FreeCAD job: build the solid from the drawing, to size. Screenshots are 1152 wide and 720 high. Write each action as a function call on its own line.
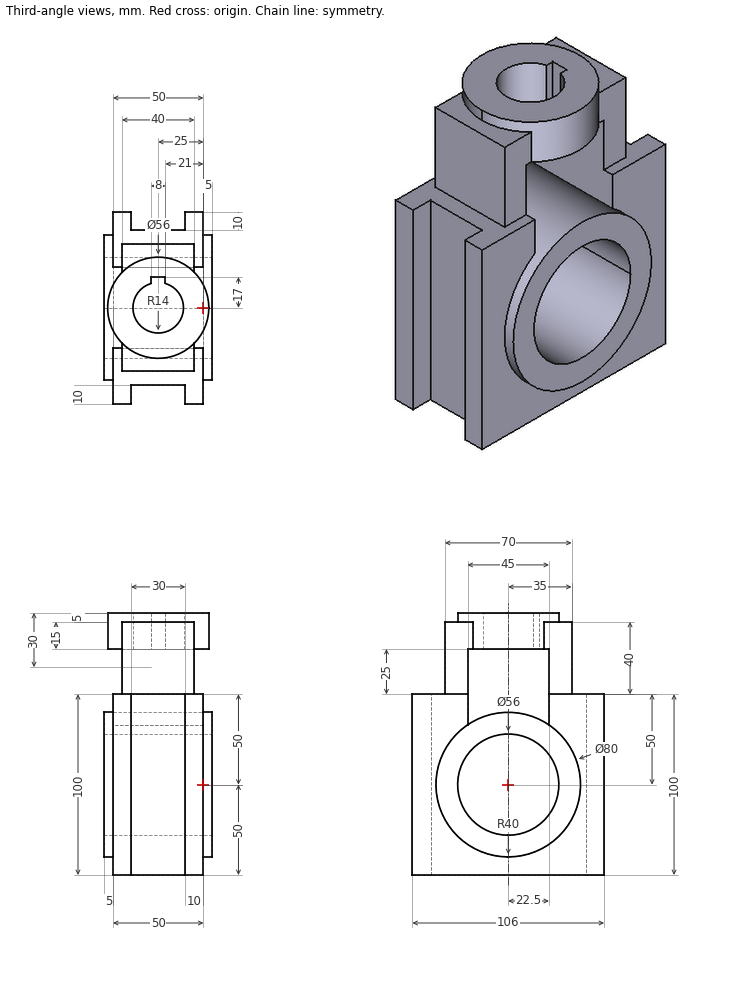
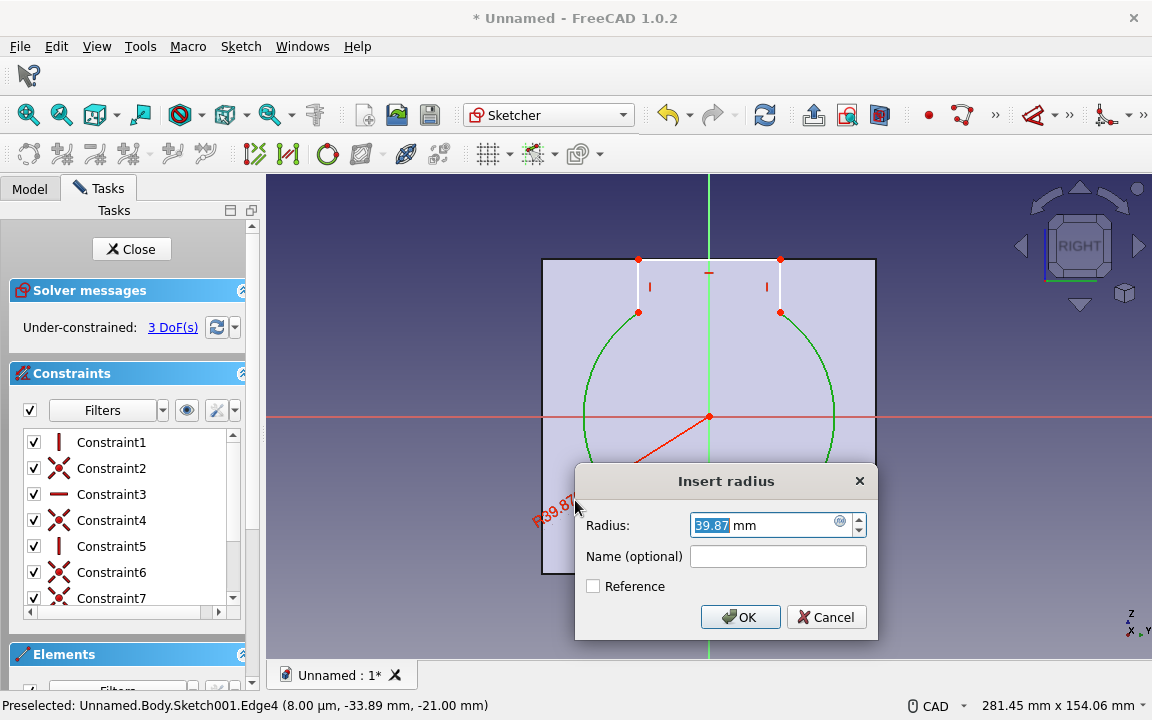
text(40)
key(Return)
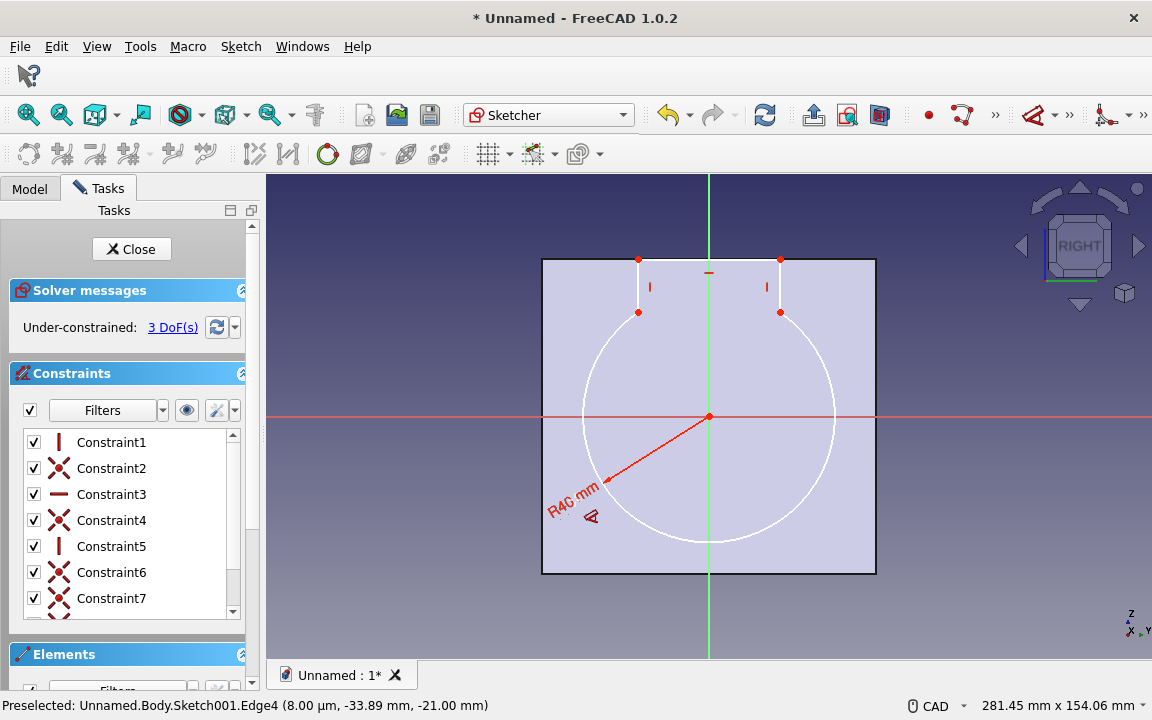
click(737, 260)
click(676, 226)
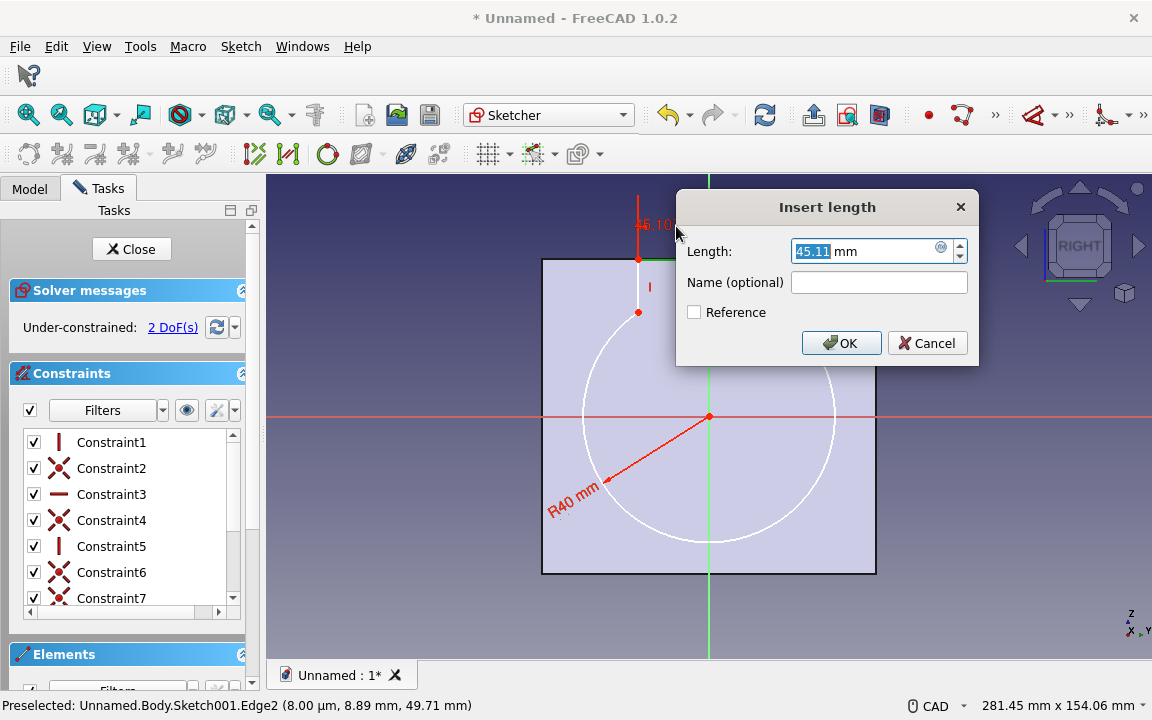
text(45)
key(Return)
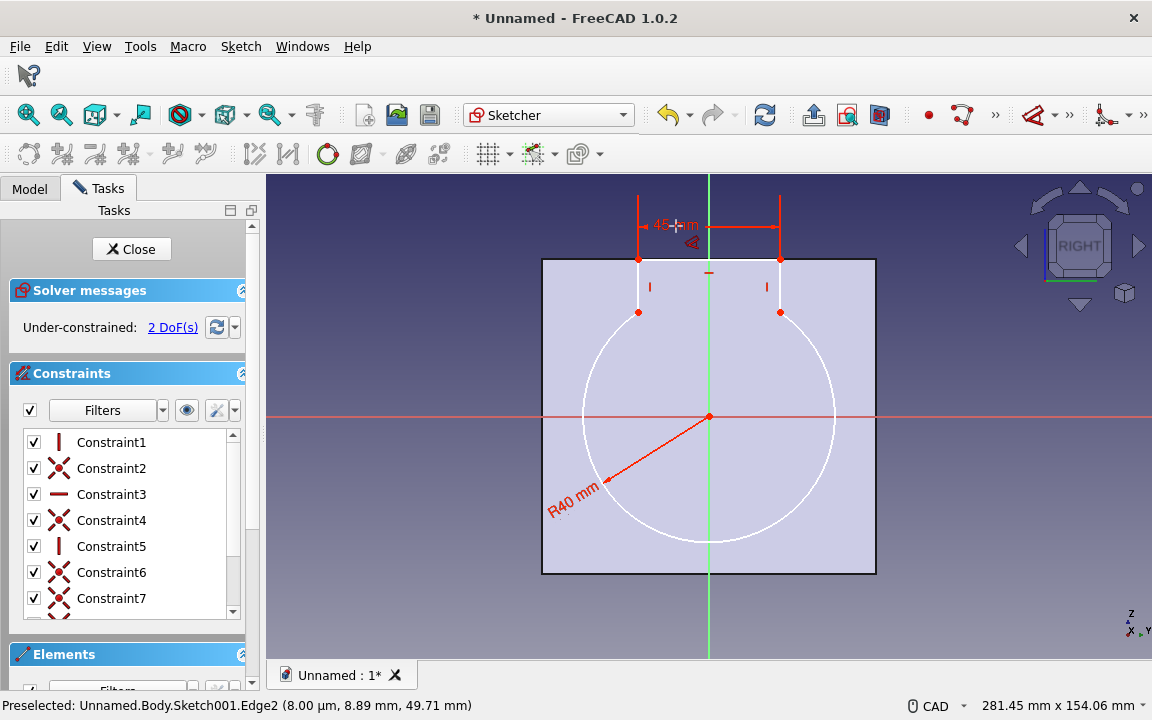
click(780, 260)
click(814, 302)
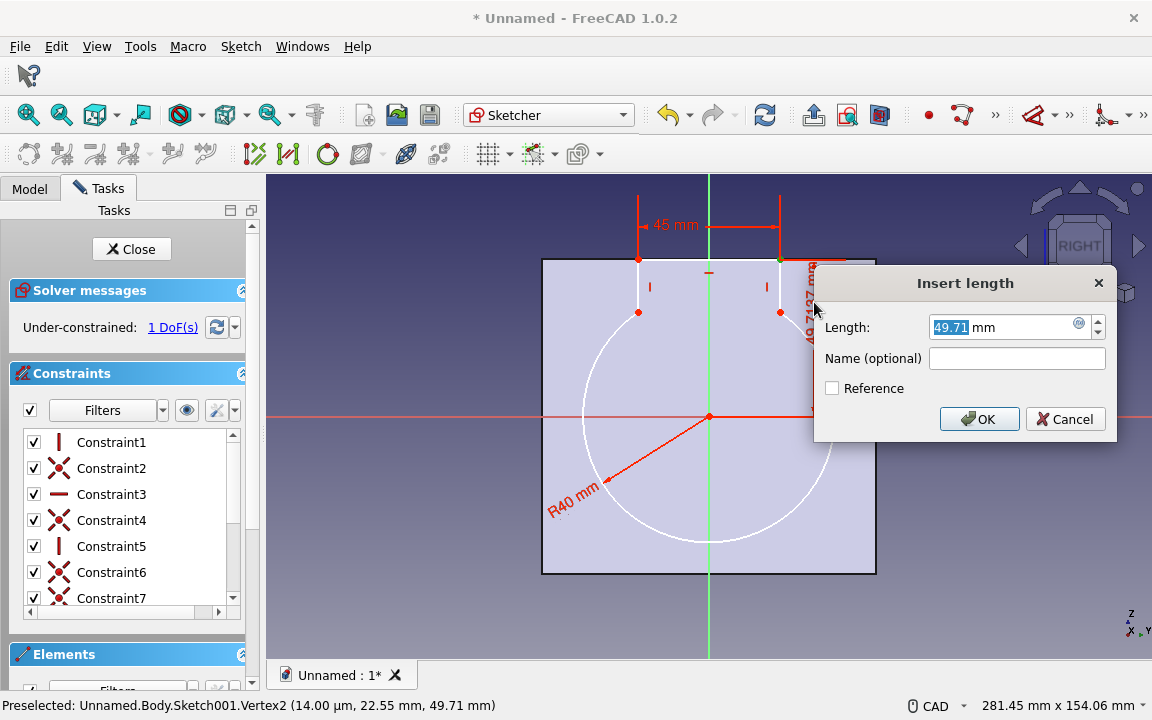
text(50)
key(Return)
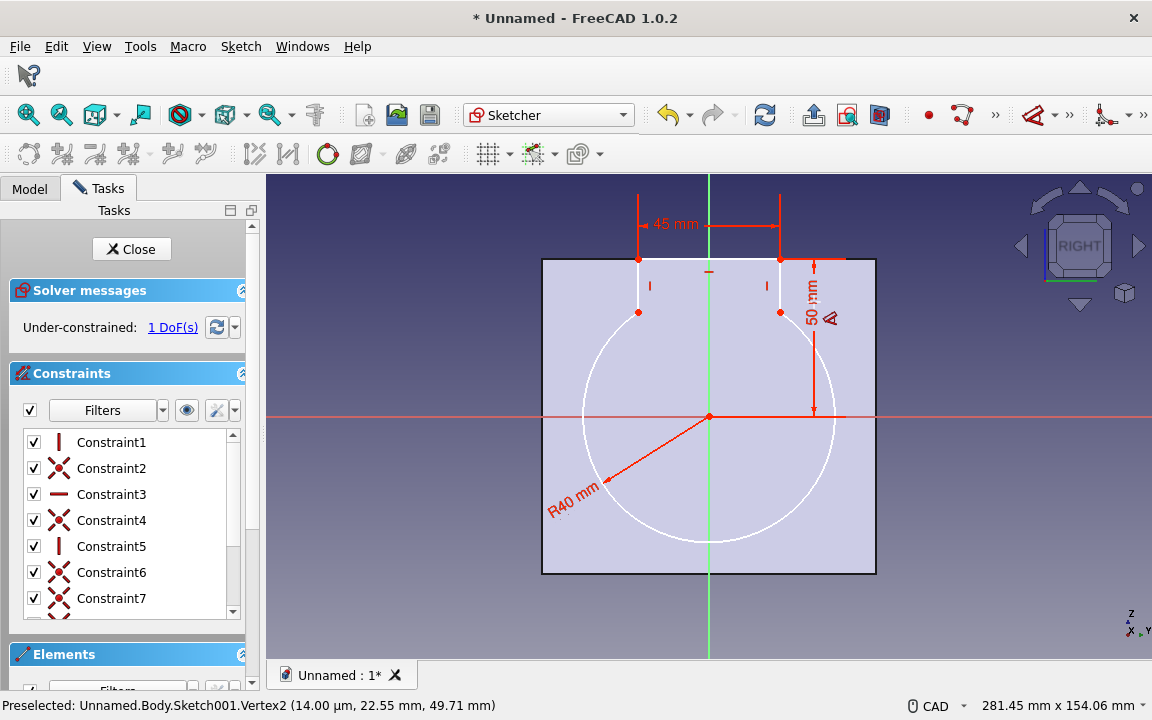
click(780, 313)
click(745, 279)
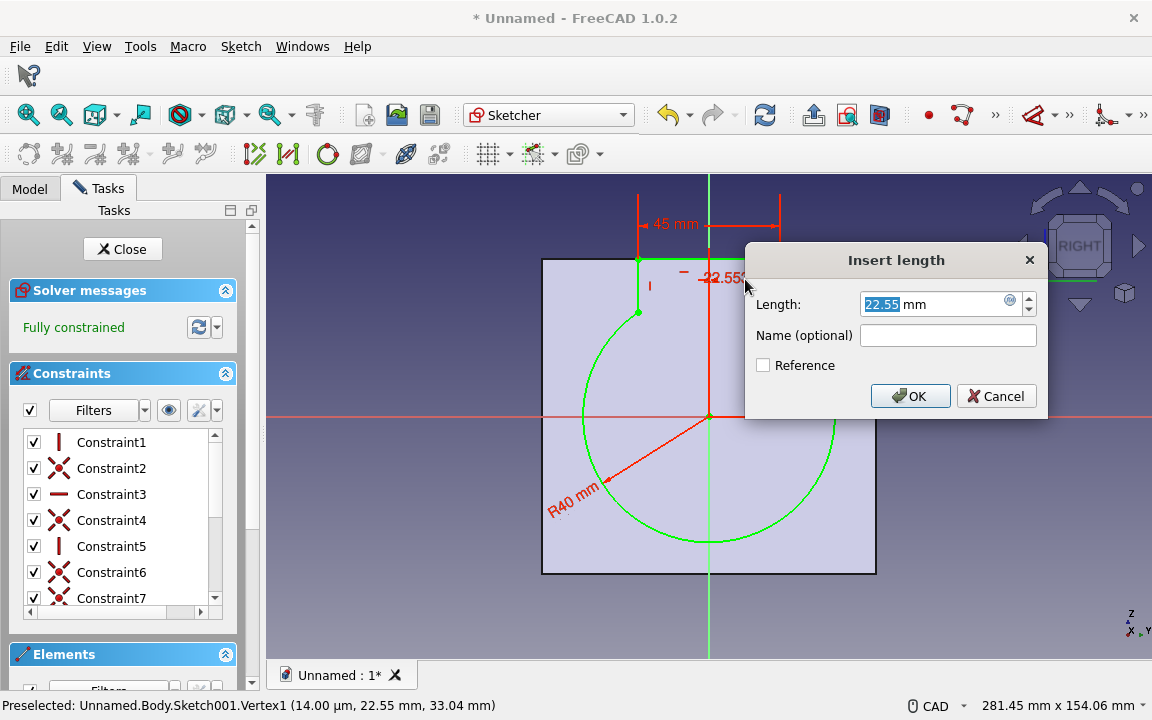
text(22.5)
key(Return)
key(Escape)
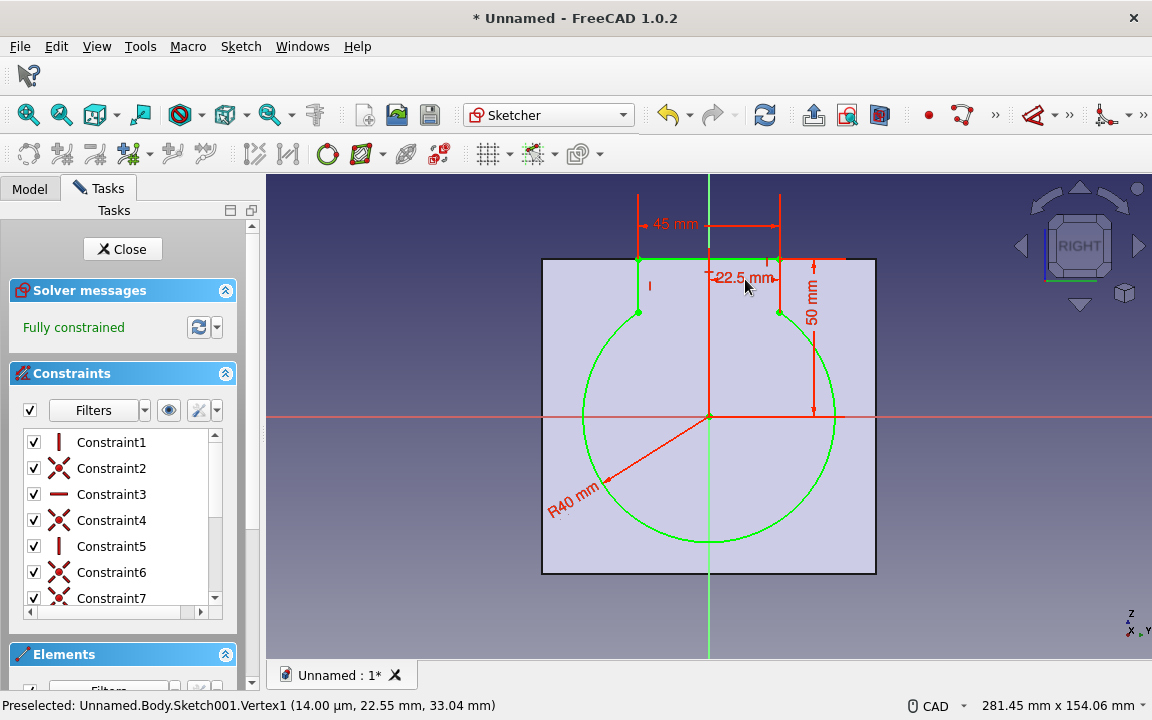
click(123, 249)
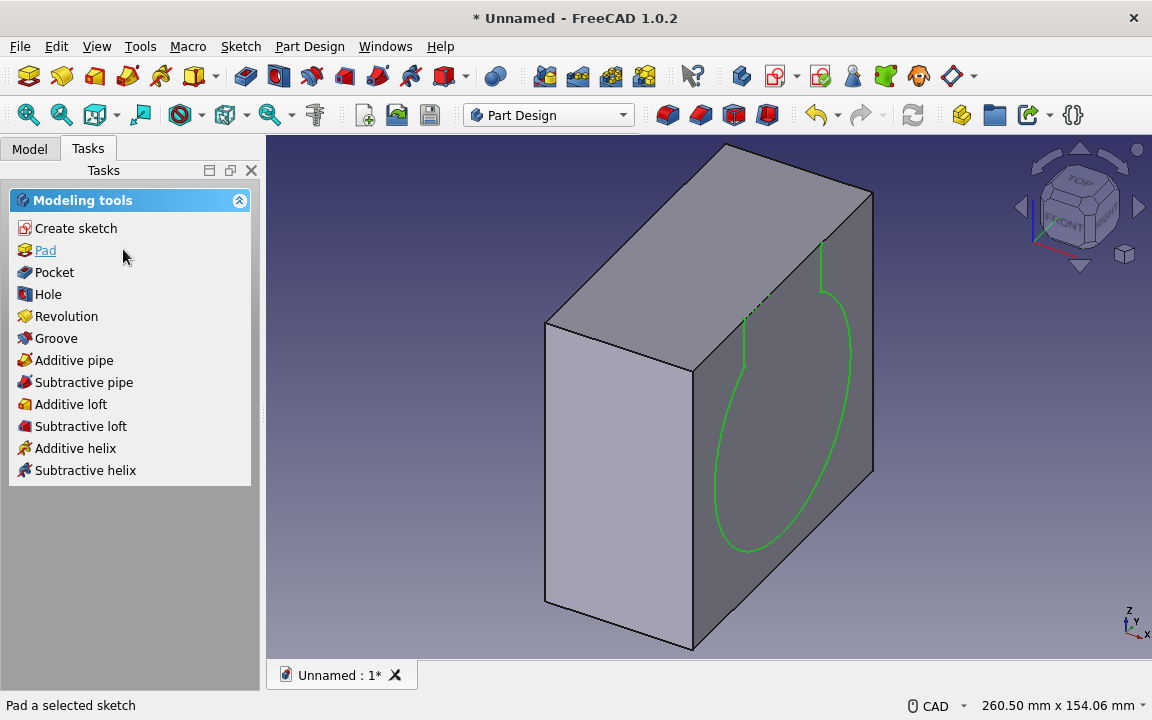
click(246, 76)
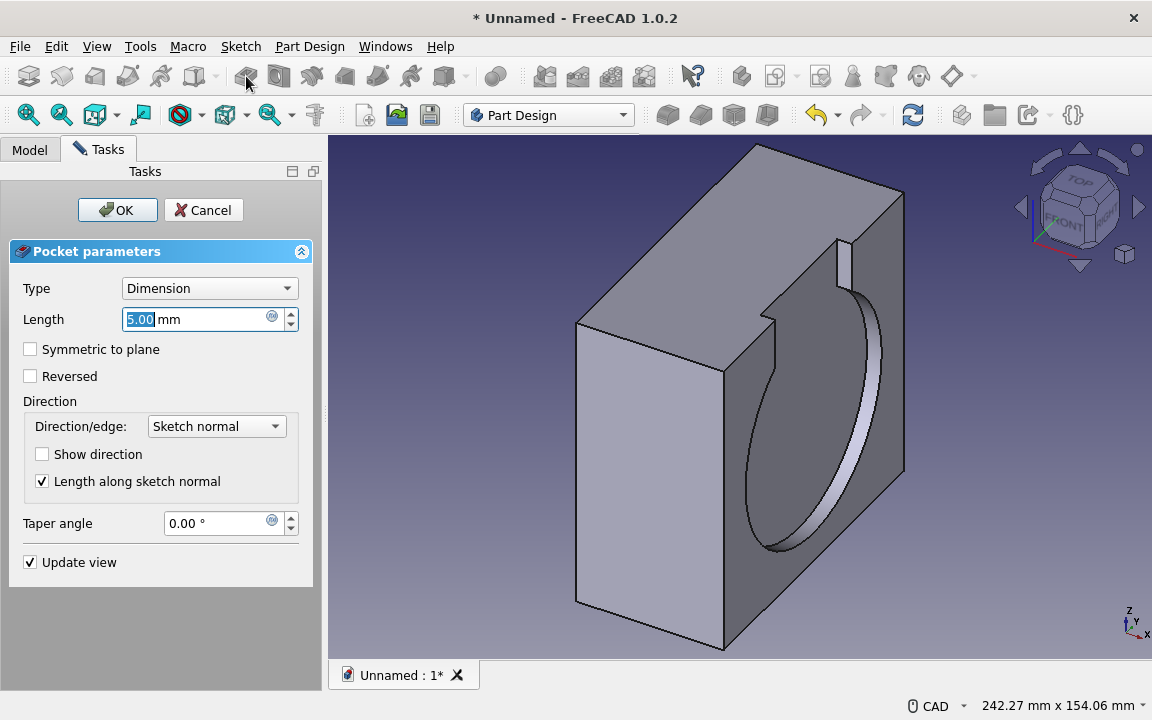
text(50)
key(Tab)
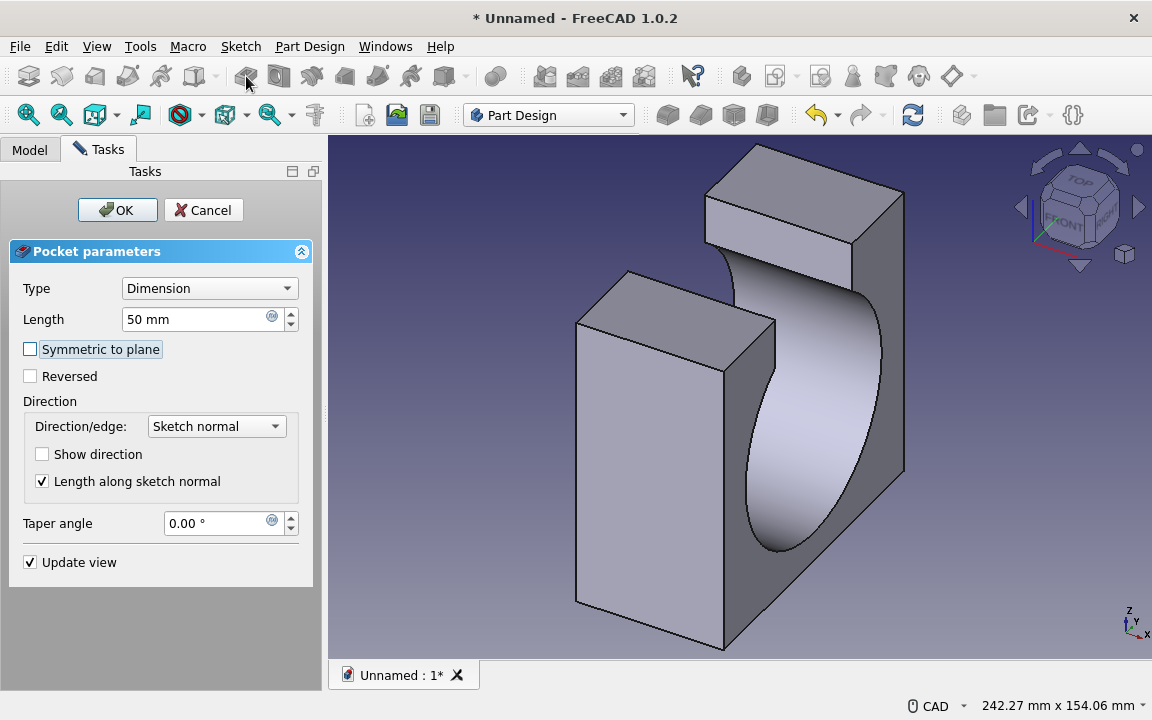
click(118, 210)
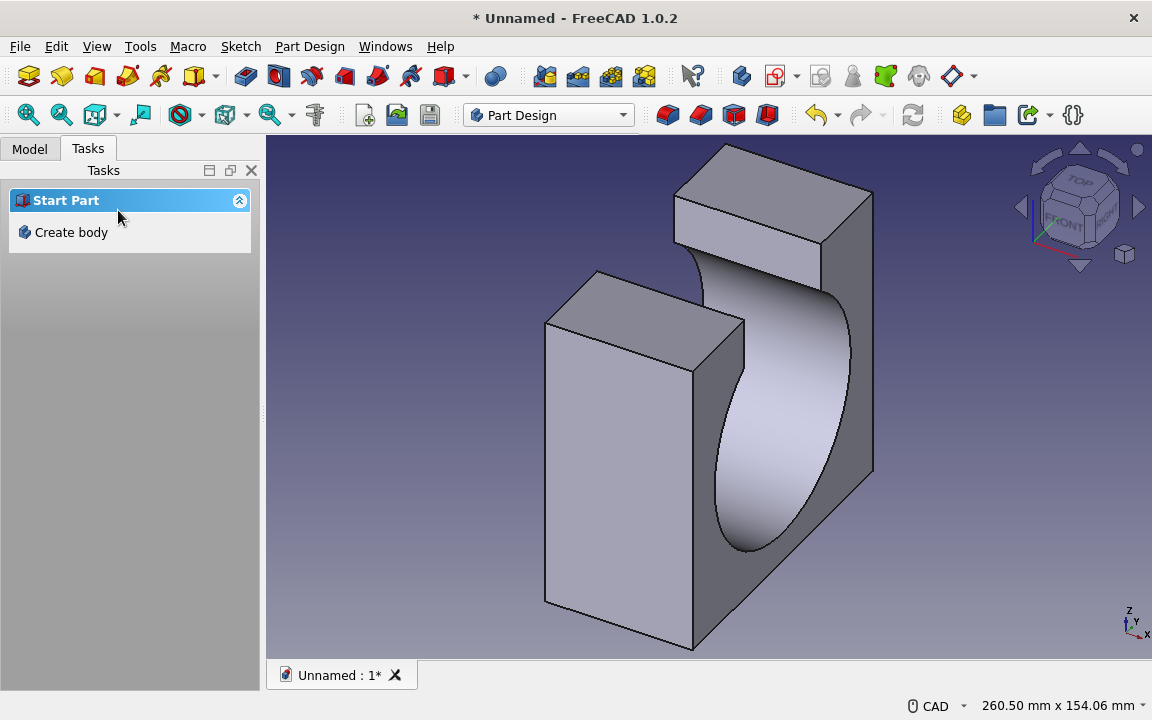
click(774, 76)